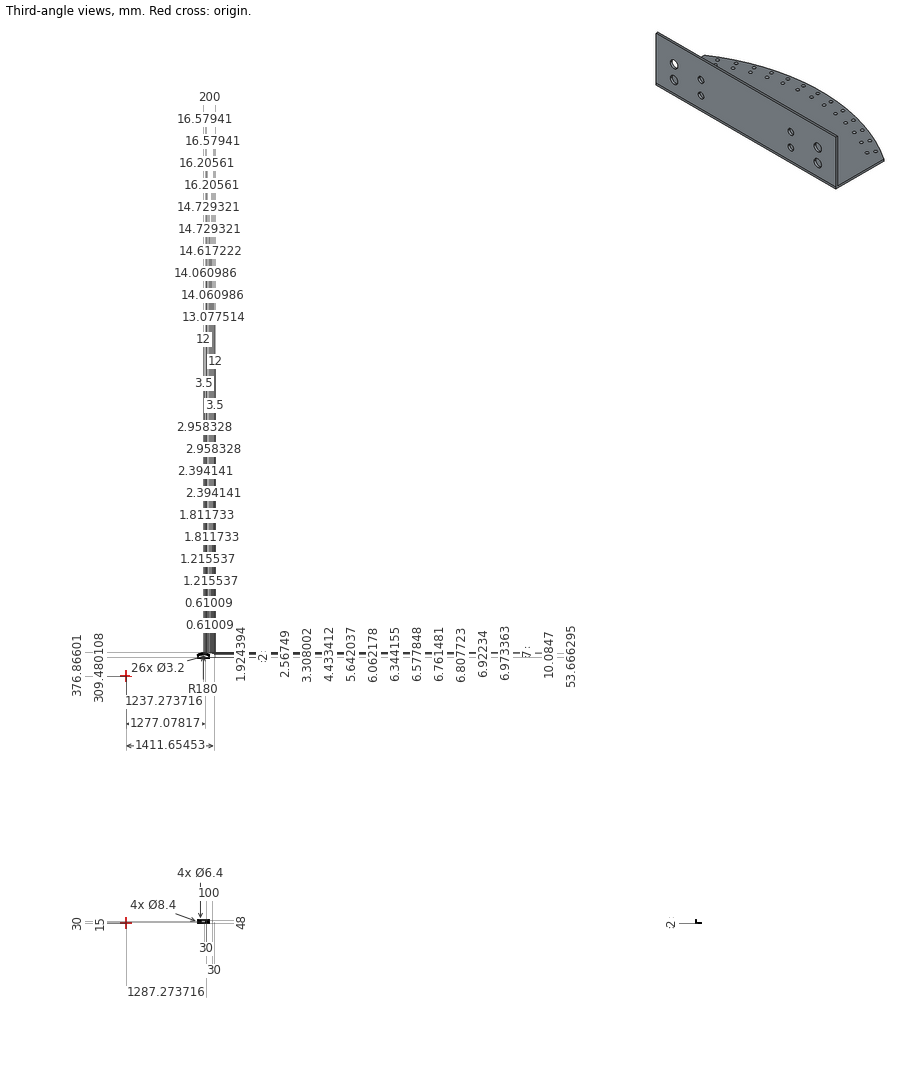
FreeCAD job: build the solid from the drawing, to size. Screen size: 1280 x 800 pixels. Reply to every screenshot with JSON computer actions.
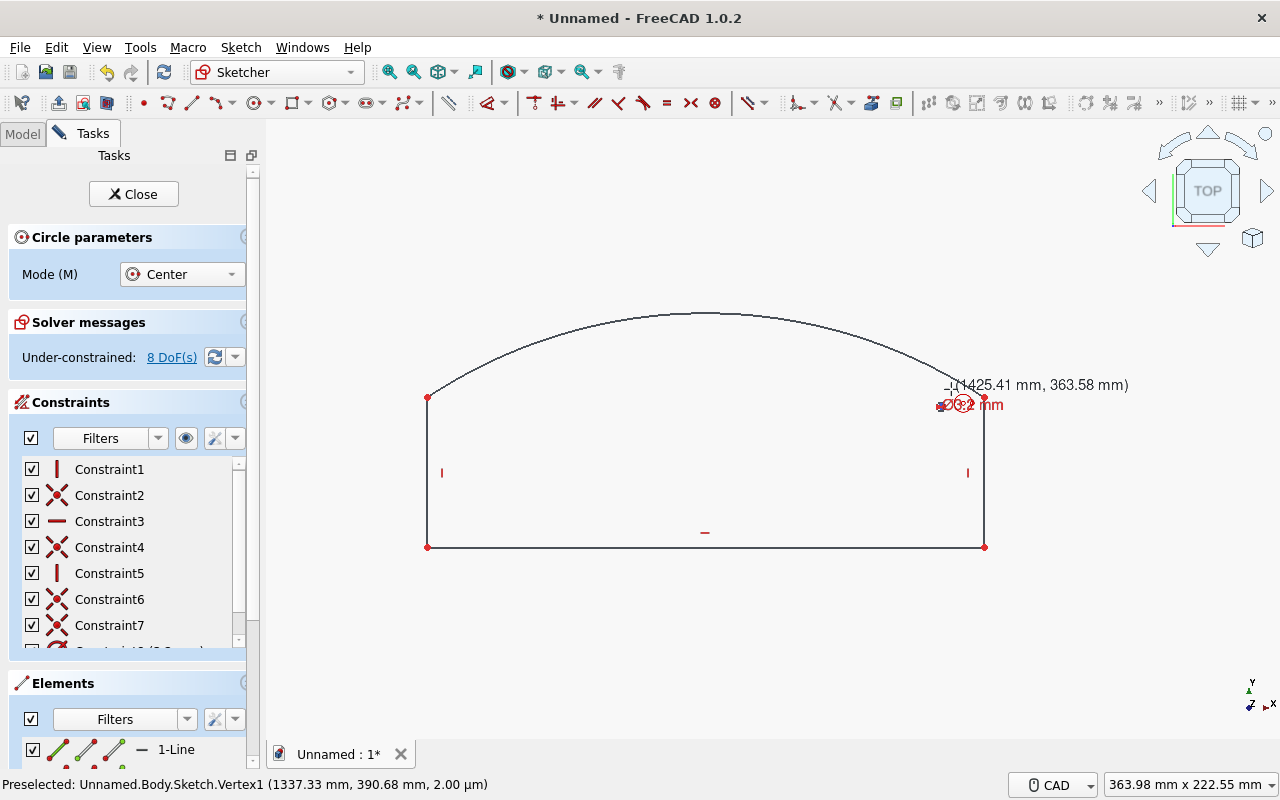
{"action": "scroll", "coordinate": [951, 389], "scroll_direction": "up", "scroll_amount": 2}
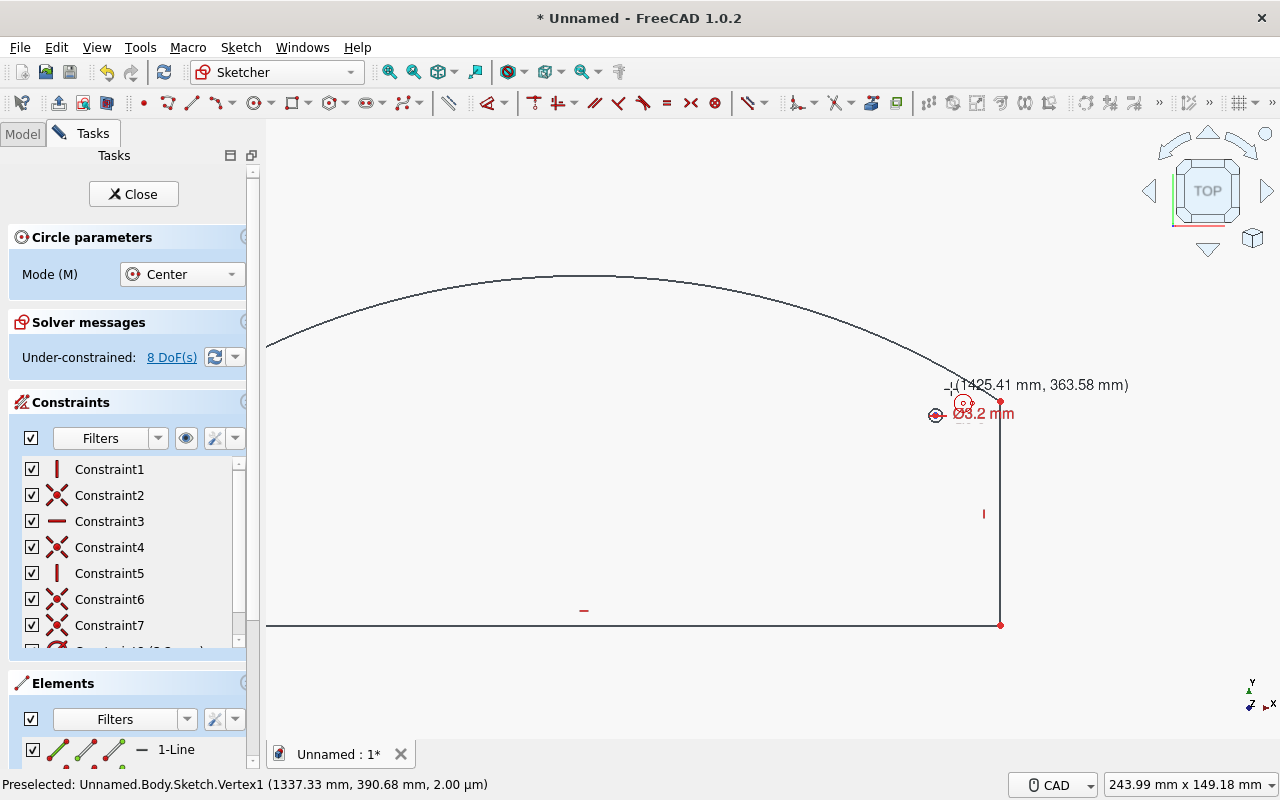
{"action": "left_click", "coordinate": [950, 389]}
{"action": "mouse_move", "coordinate": [945, 384]}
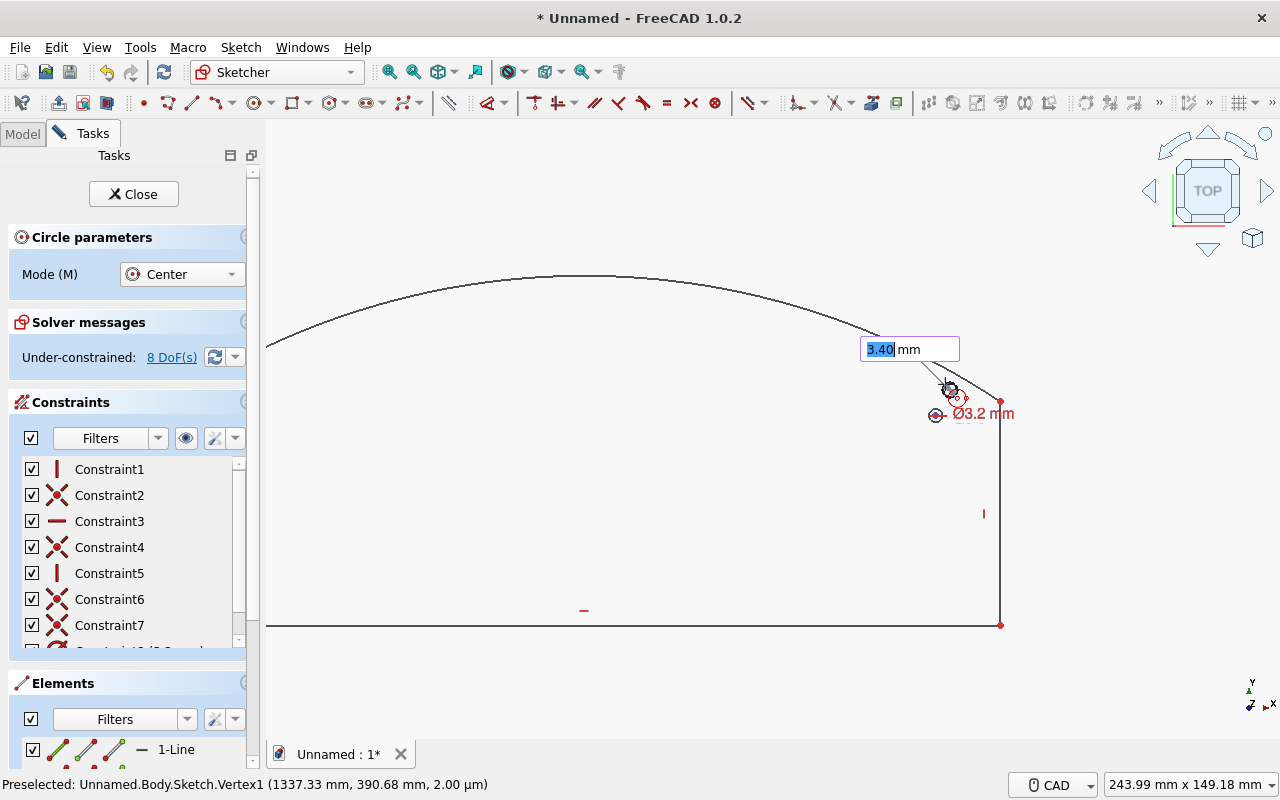
{"action": "type", "text": "3.2"}
{"action": "key", "text": "Return"}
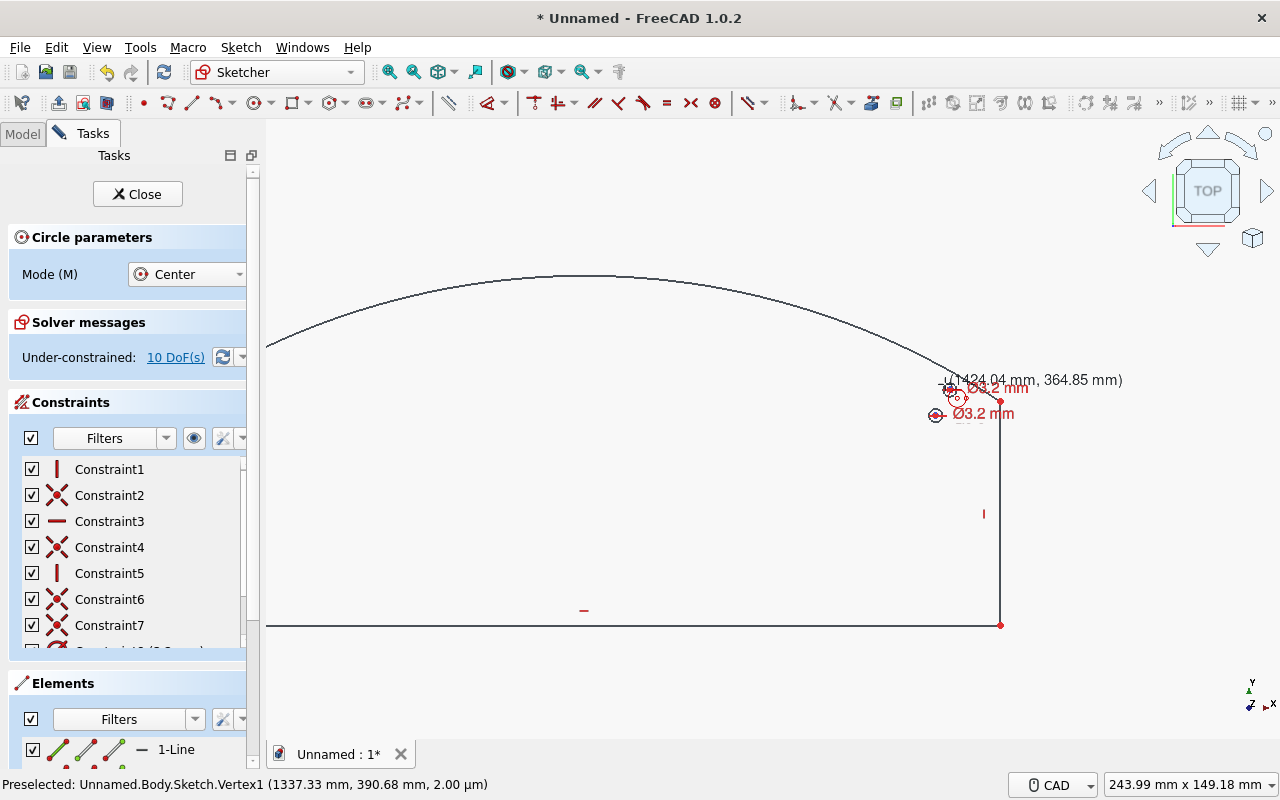
{"action": "scroll", "coordinate": [881, 386], "scroll_direction": "up", "scroll_amount": 7}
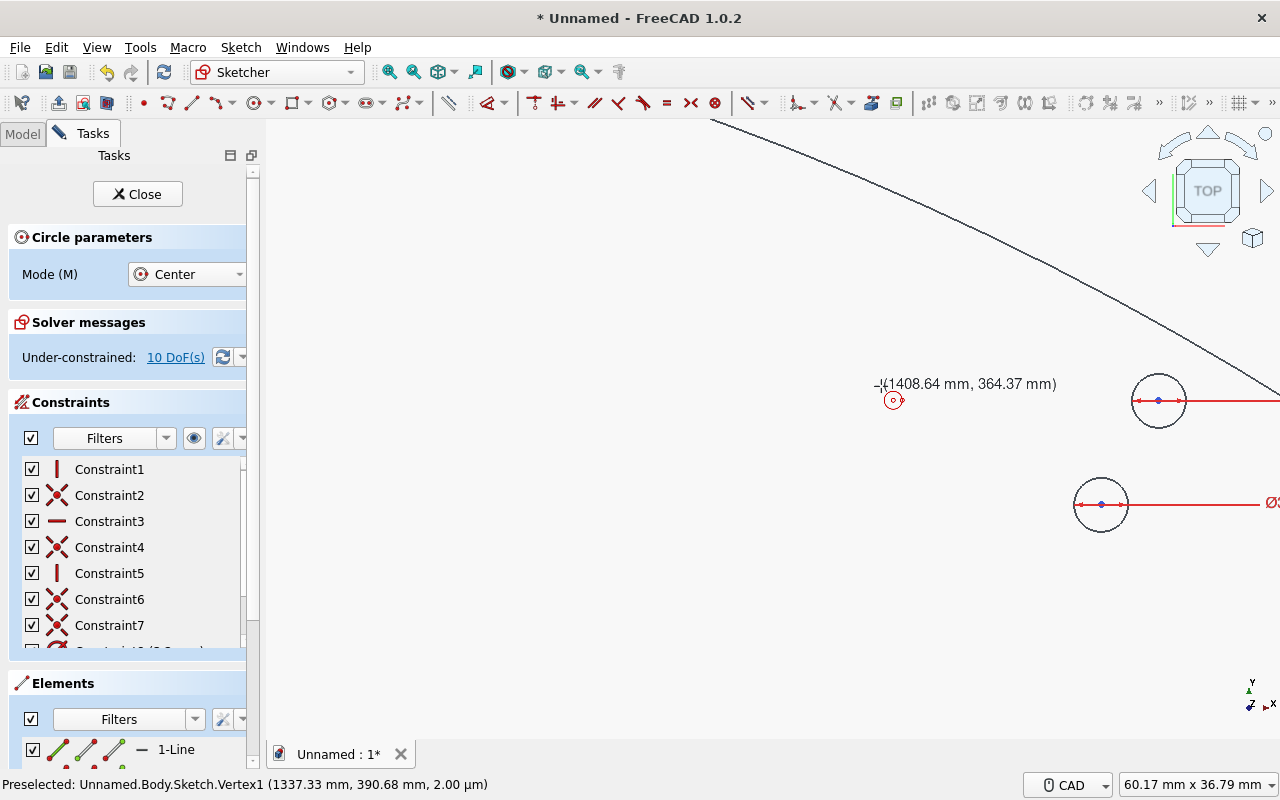
{"action": "scroll", "coordinate": [908, 387], "scroll_direction": "down", "scroll_amount": 9}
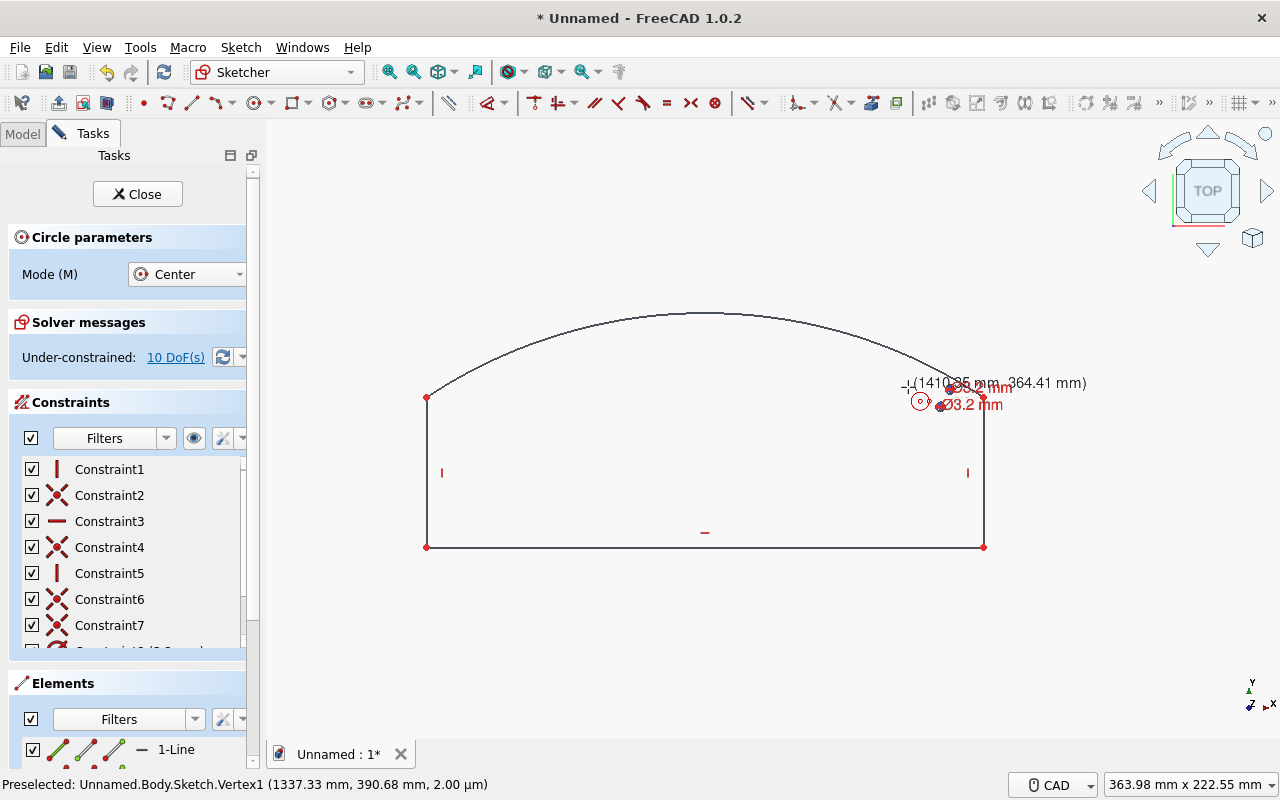
{"action": "left_click", "coordinate": [904, 387]}
{"action": "mouse_move", "coordinate": [907, 384]}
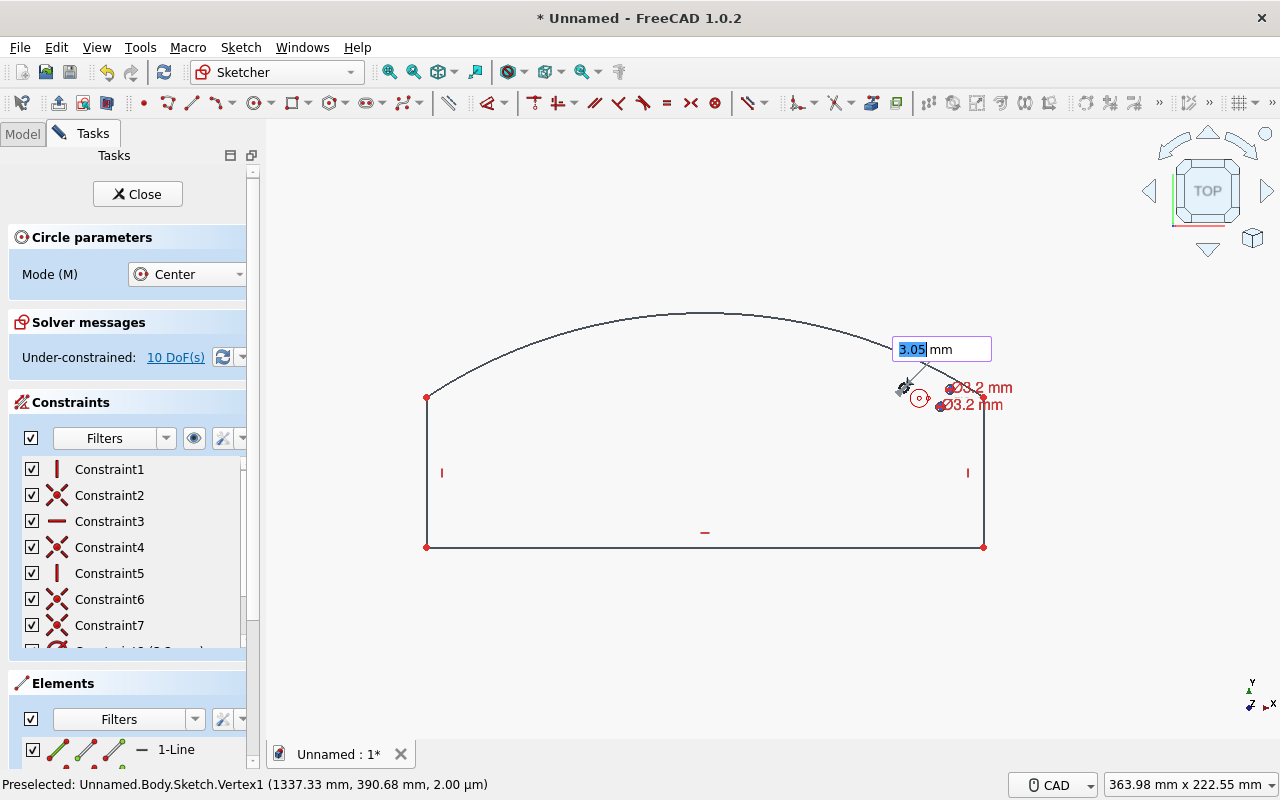
{"action": "type", "text": "3.2"}
{"action": "key", "text": "Return"}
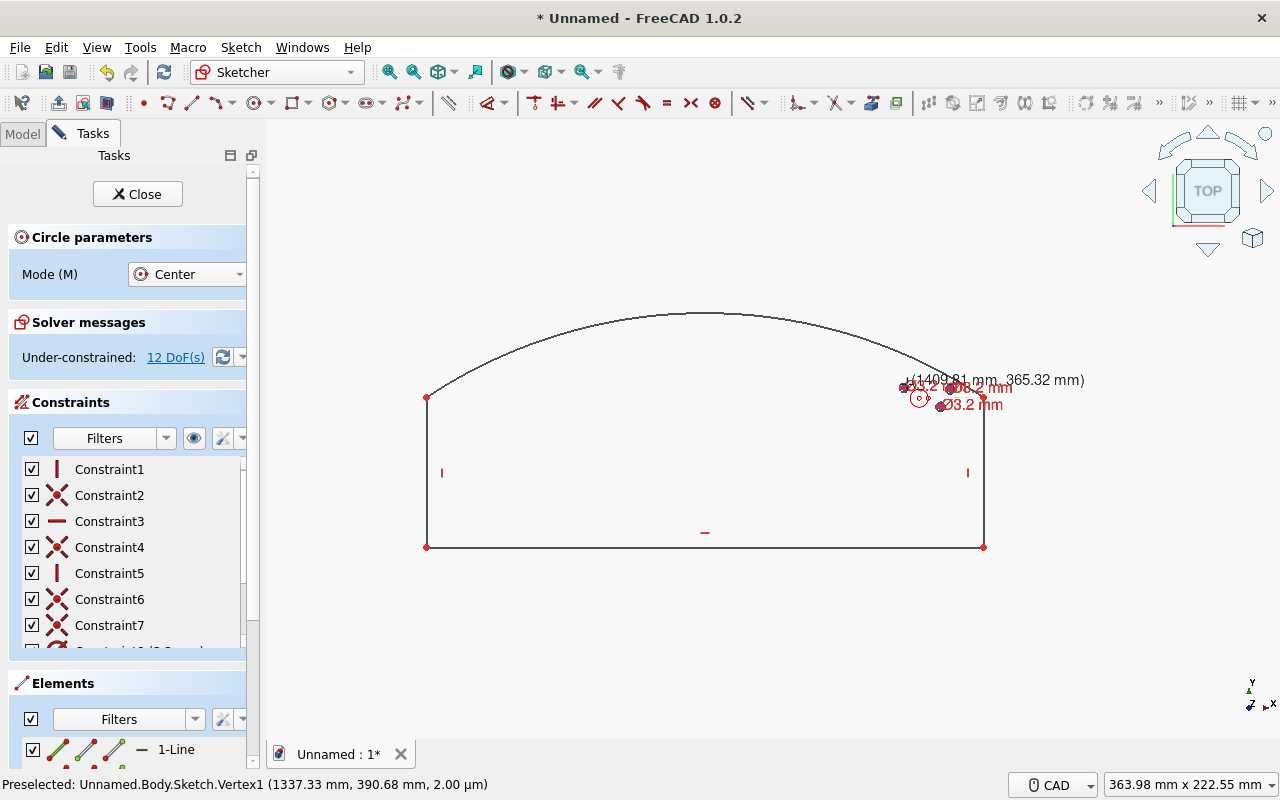
{"action": "scroll", "coordinate": [912, 369], "scroll_direction": "up", "scroll_amount": 9}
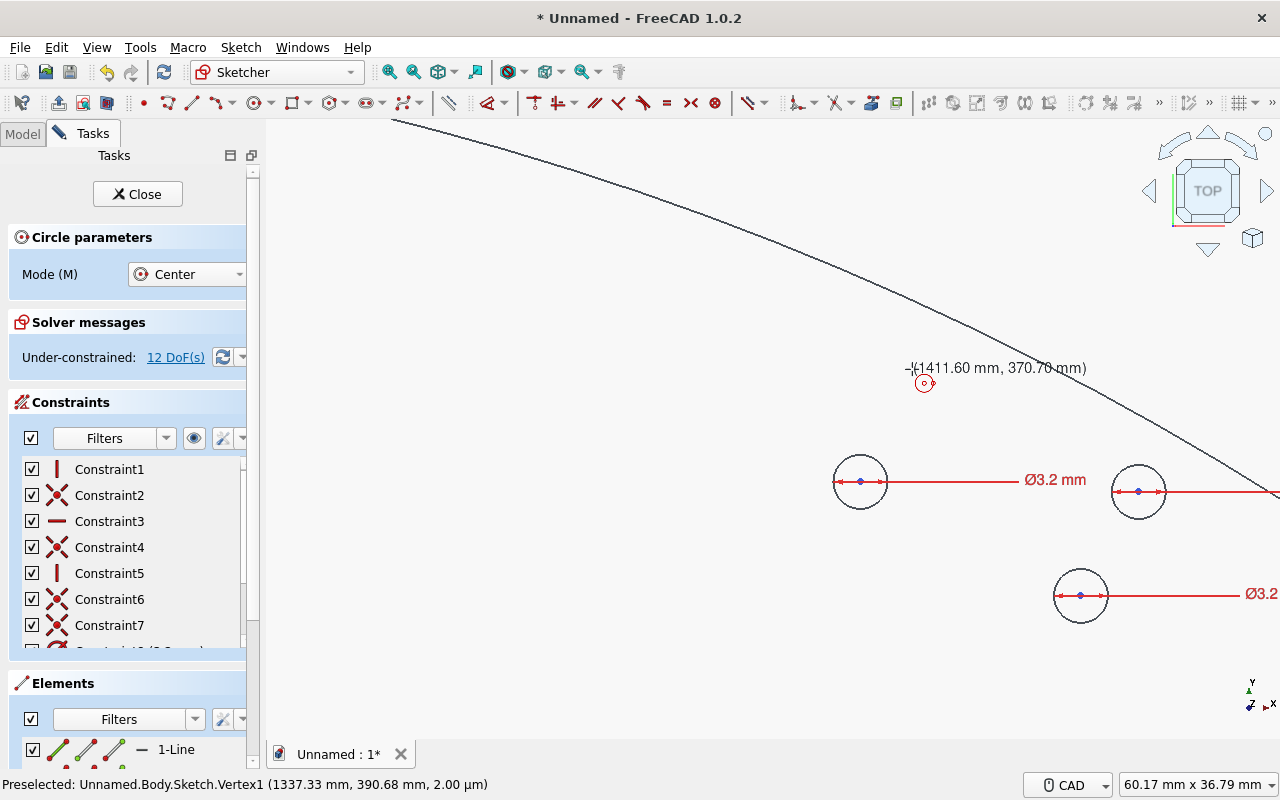
{"action": "scroll", "coordinate": [912, 369], "scroll_direction": "down", "scroll_amount": 9}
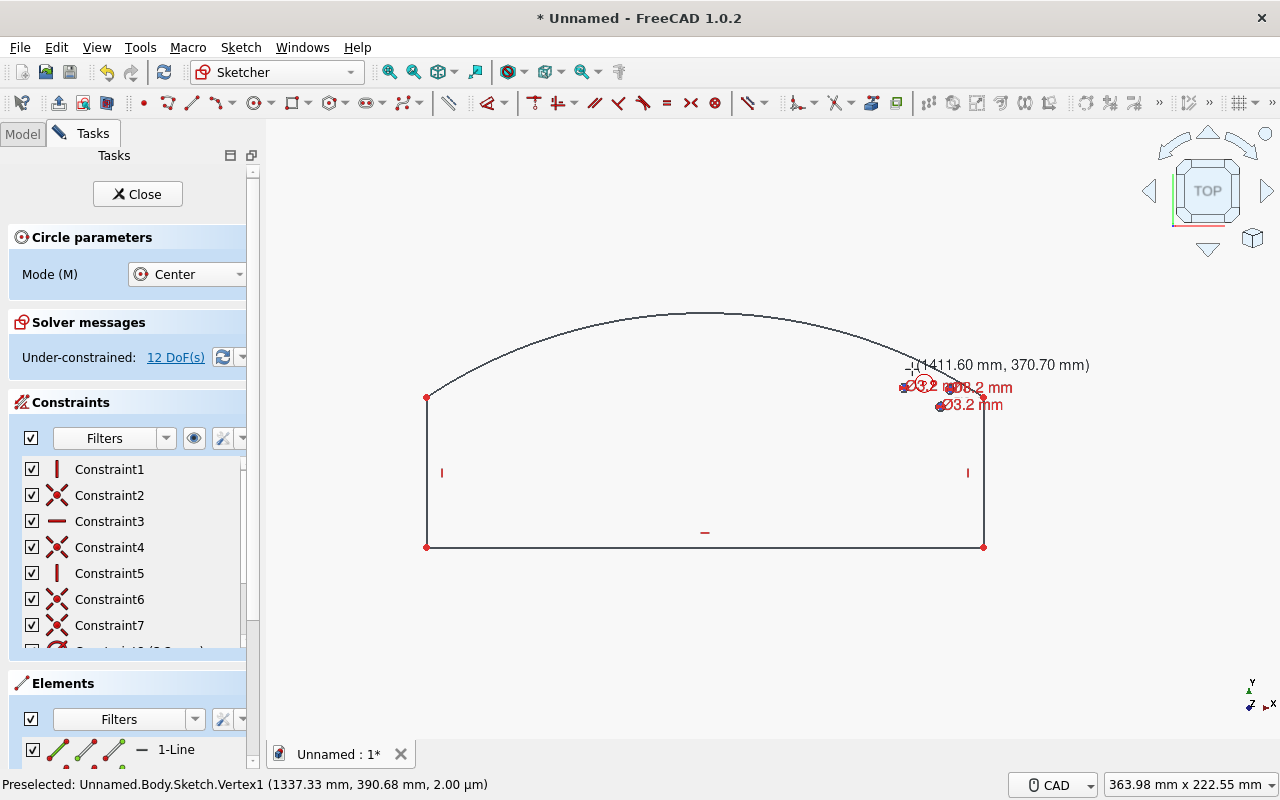
{"action": "scroll", "coordinate": [912, 369], "scroll_direction": "up", "scroll_amount": 2}